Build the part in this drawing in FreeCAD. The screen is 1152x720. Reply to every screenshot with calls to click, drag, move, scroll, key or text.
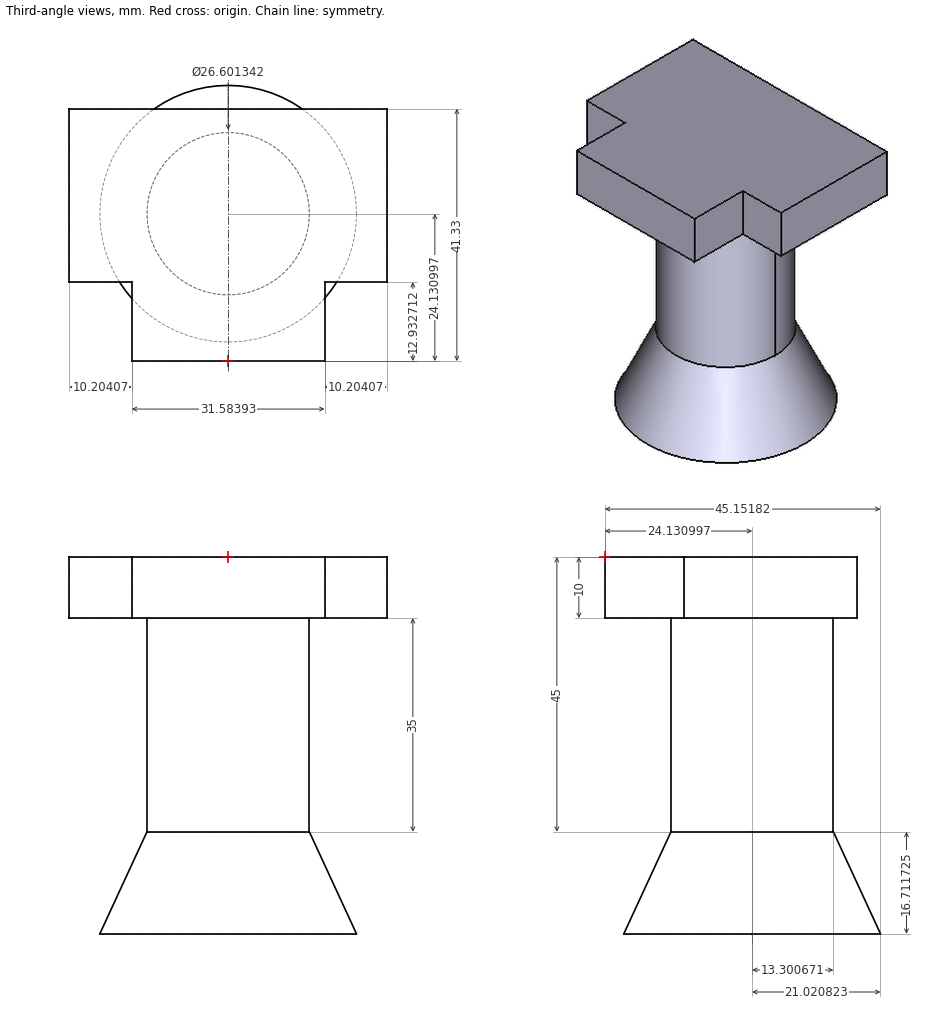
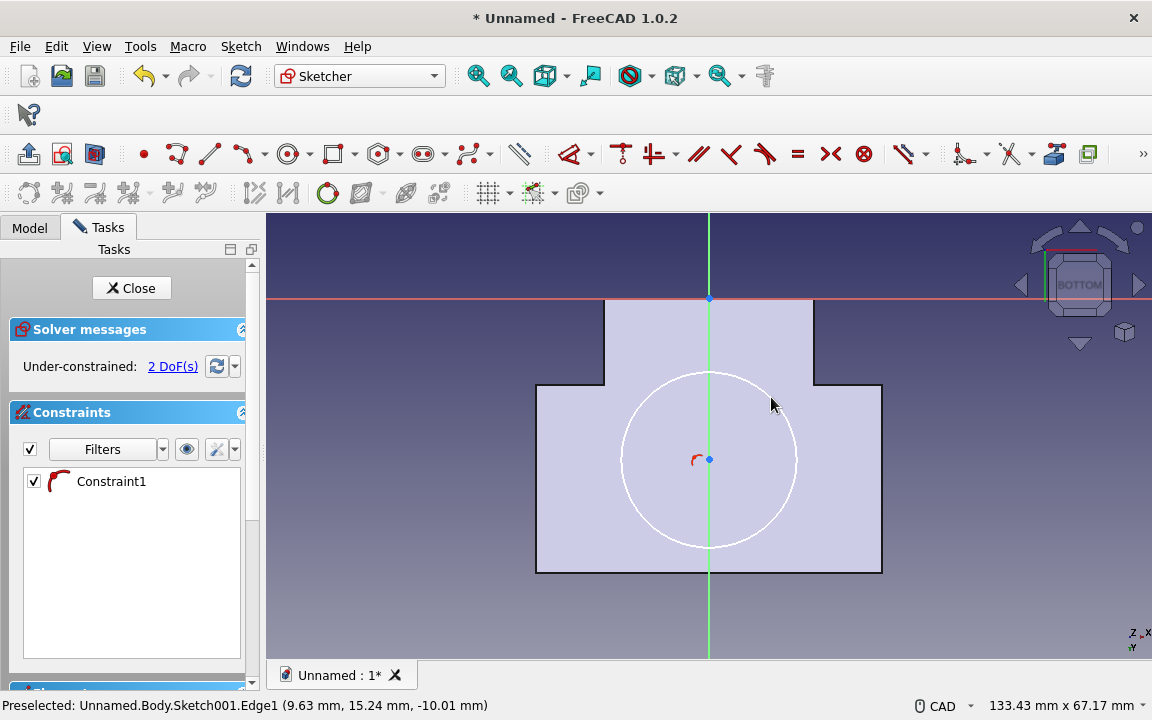
click(568, 154)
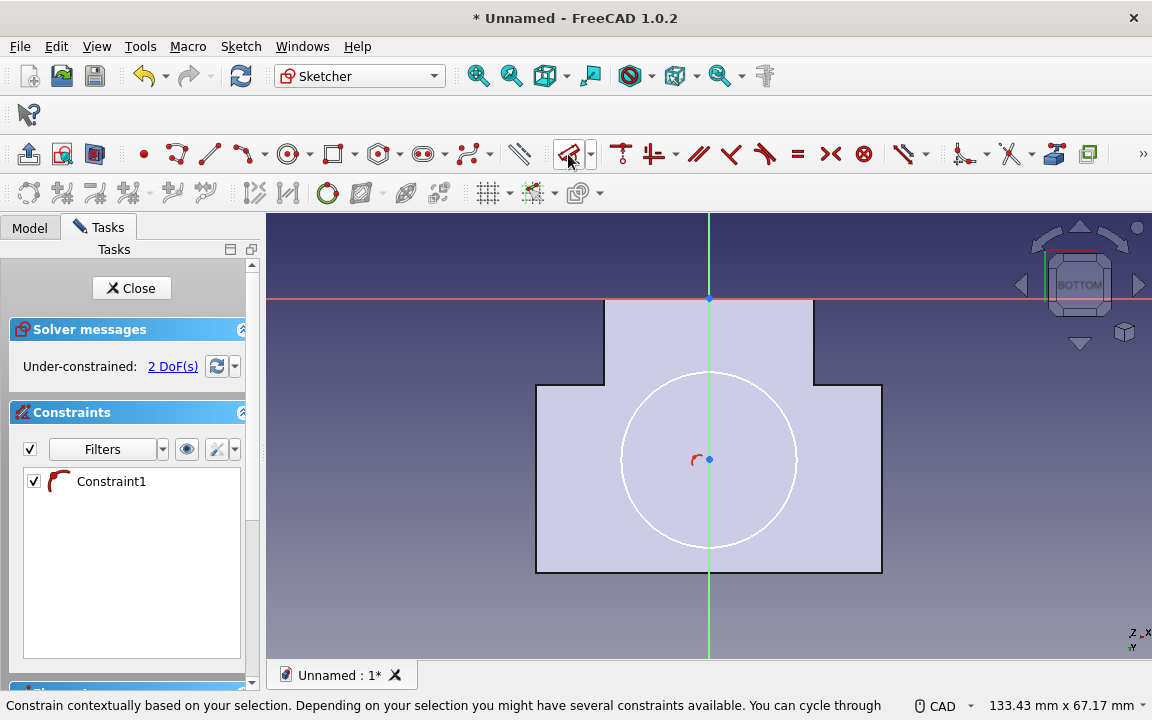
click(771, 398)
click(794, 375)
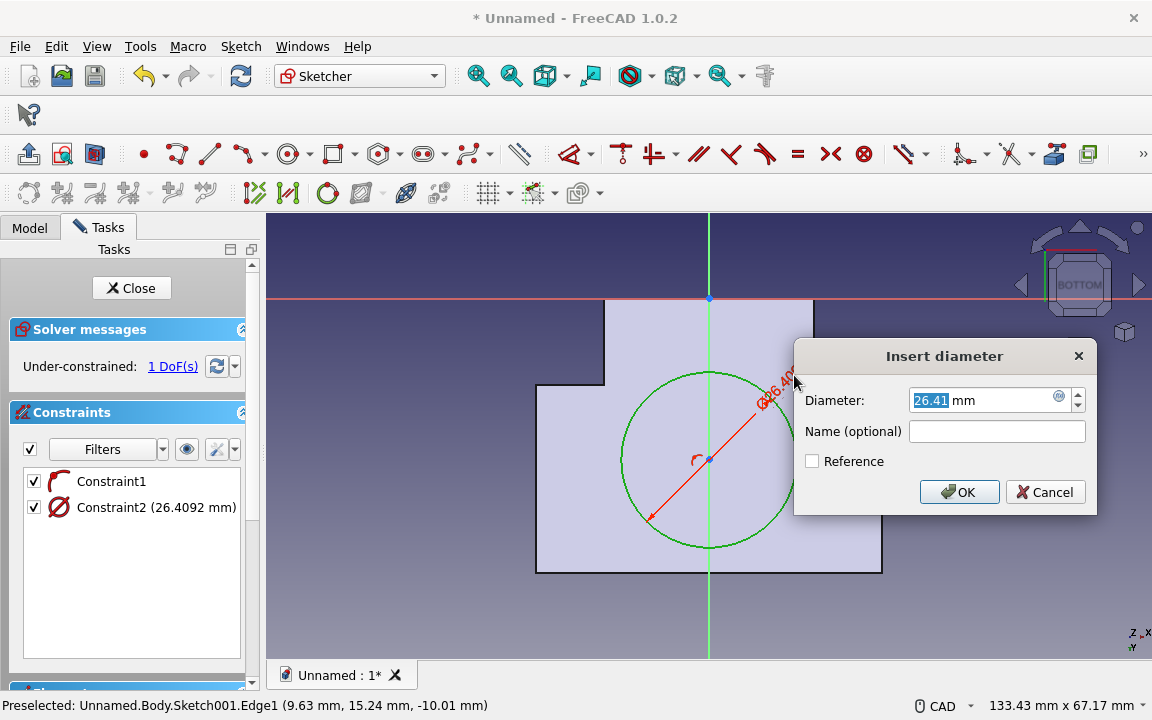
text(26.601342)
key(Return)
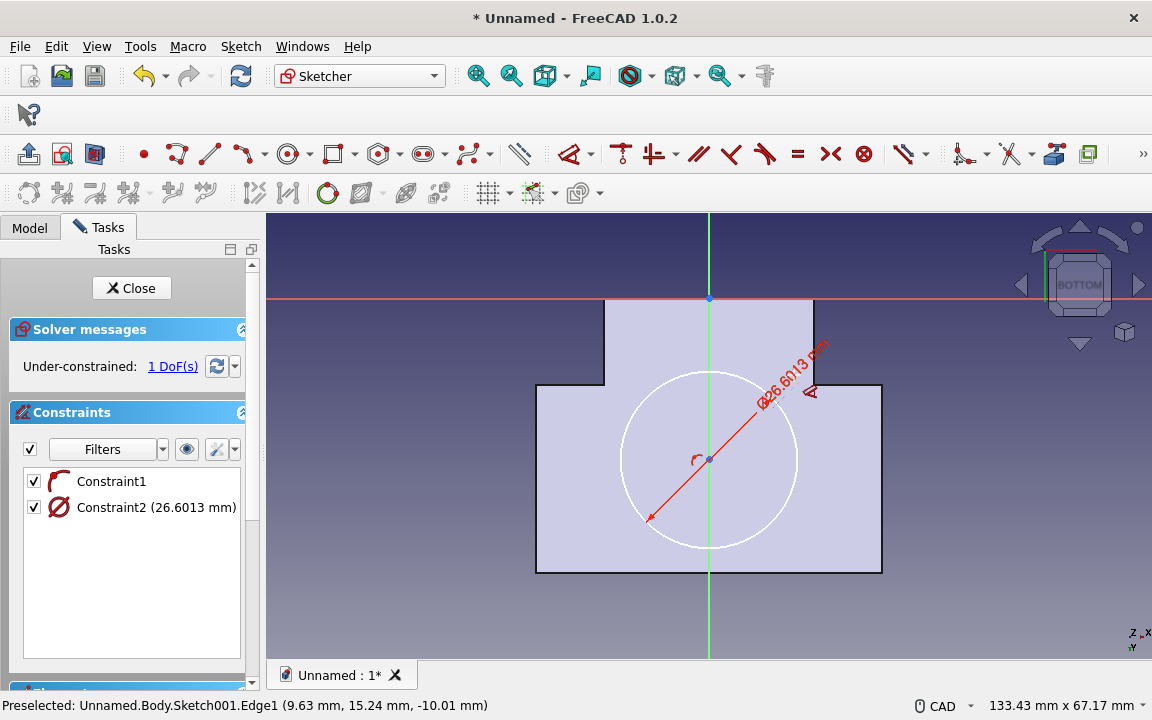
click(709, 460)
click(743, 342)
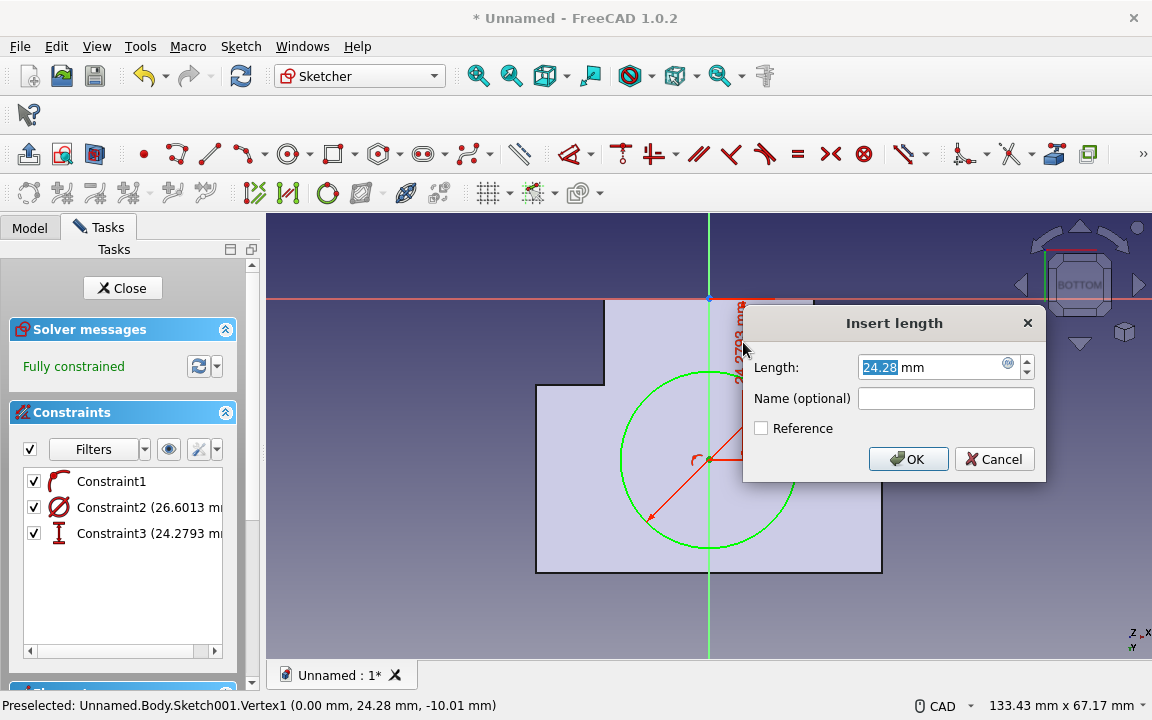
text(24.130997)
key(Return)
key(Escape)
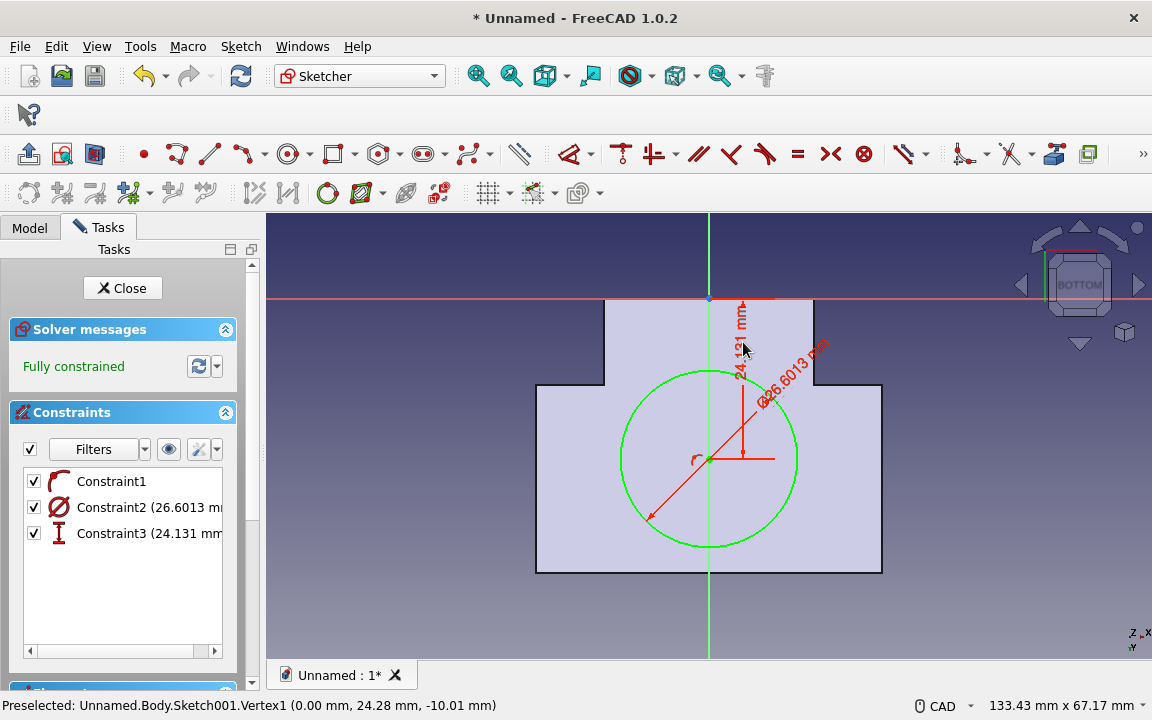
click(123, 288)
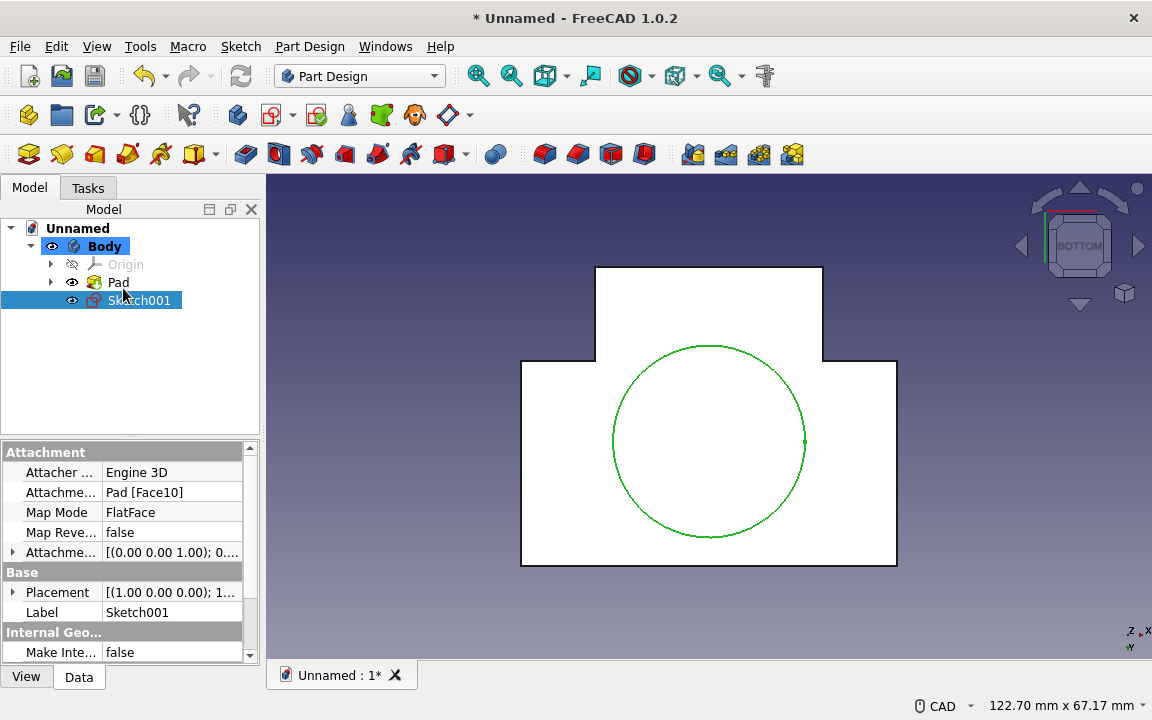
click(29, 154)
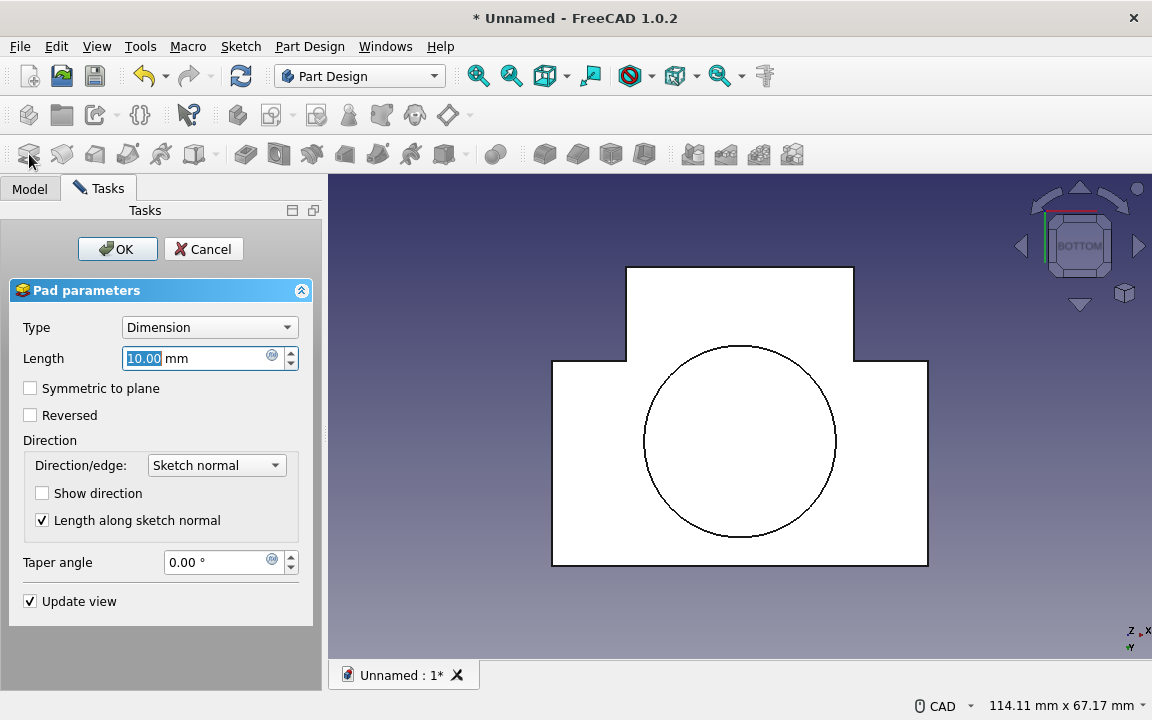
text(35)
key(Tab)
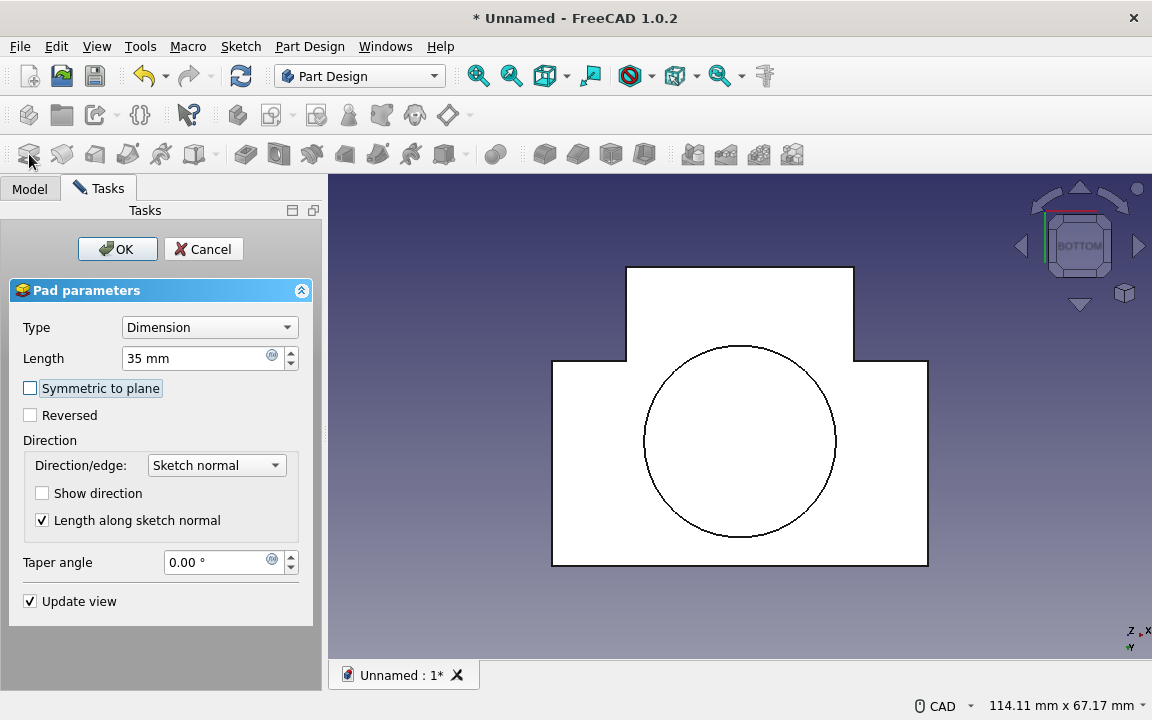
click(118, 249)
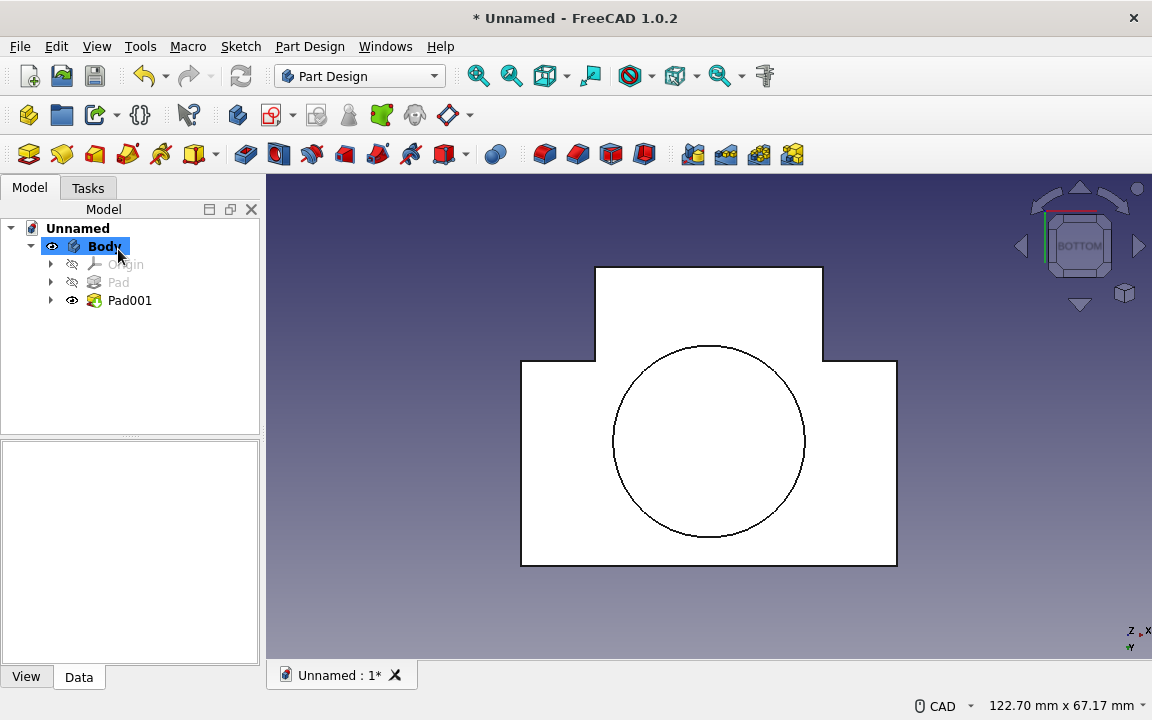
click(270, 116)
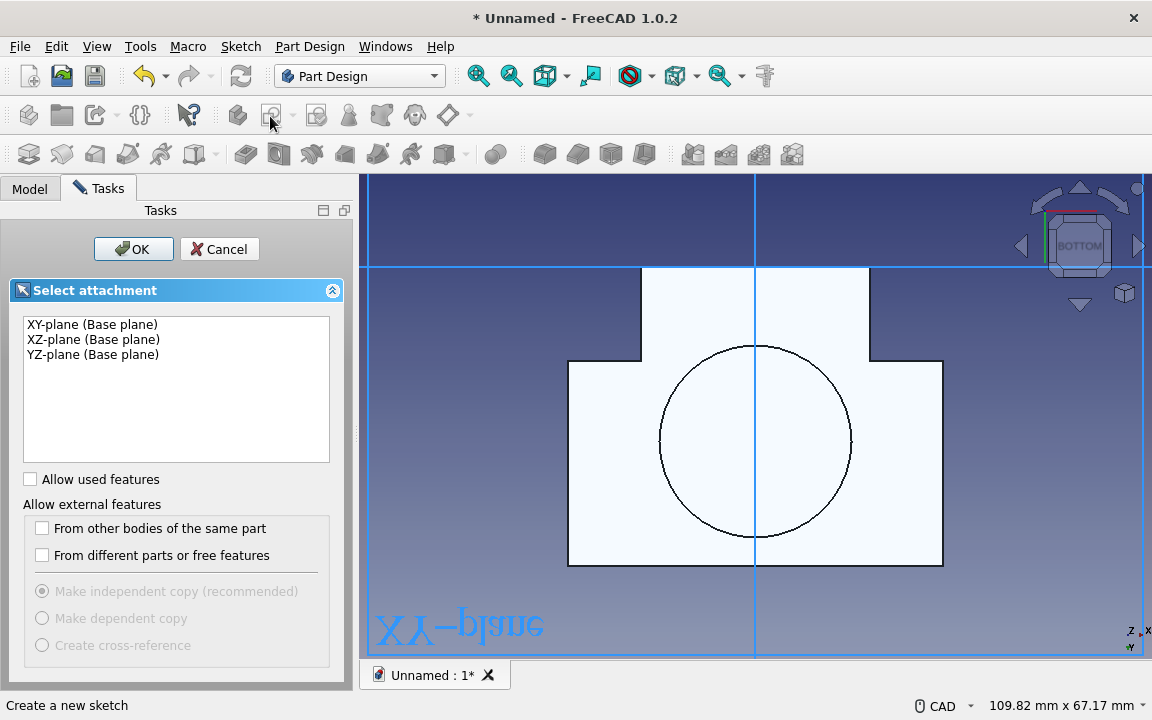
click(84, 354)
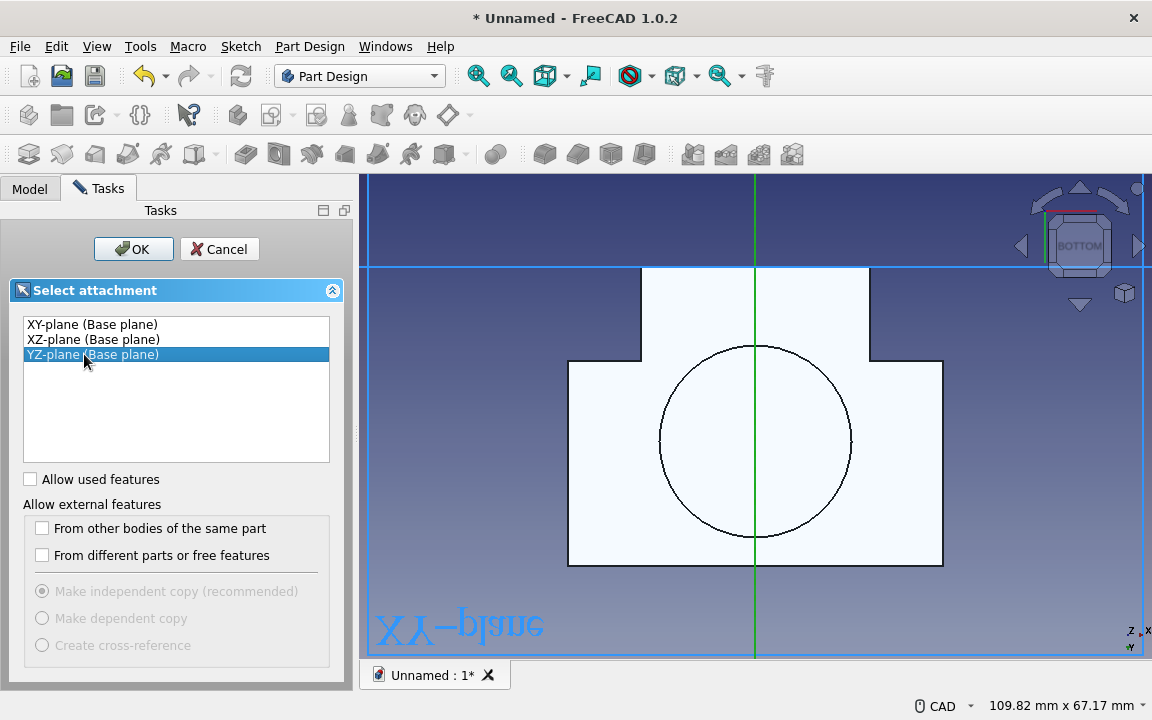
click(134, 249)